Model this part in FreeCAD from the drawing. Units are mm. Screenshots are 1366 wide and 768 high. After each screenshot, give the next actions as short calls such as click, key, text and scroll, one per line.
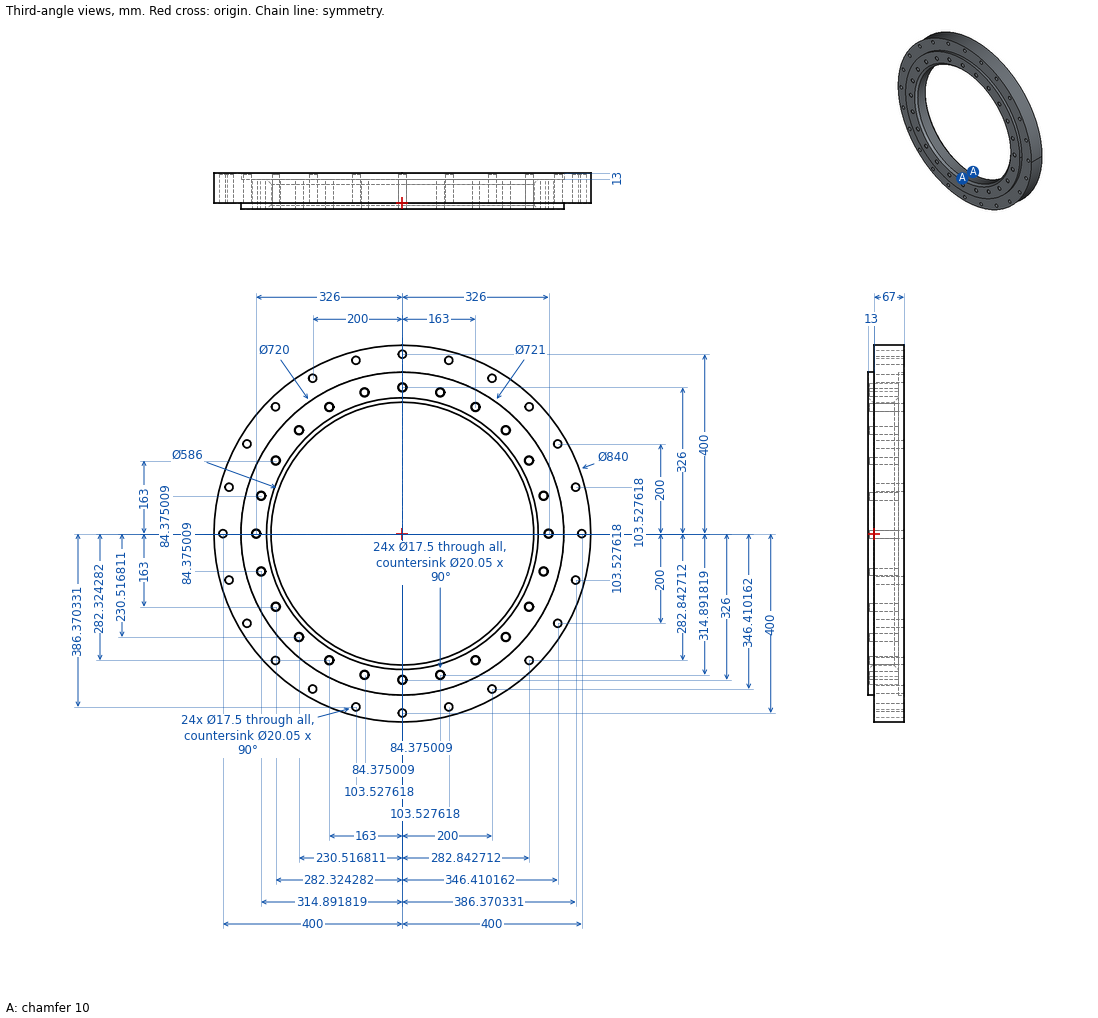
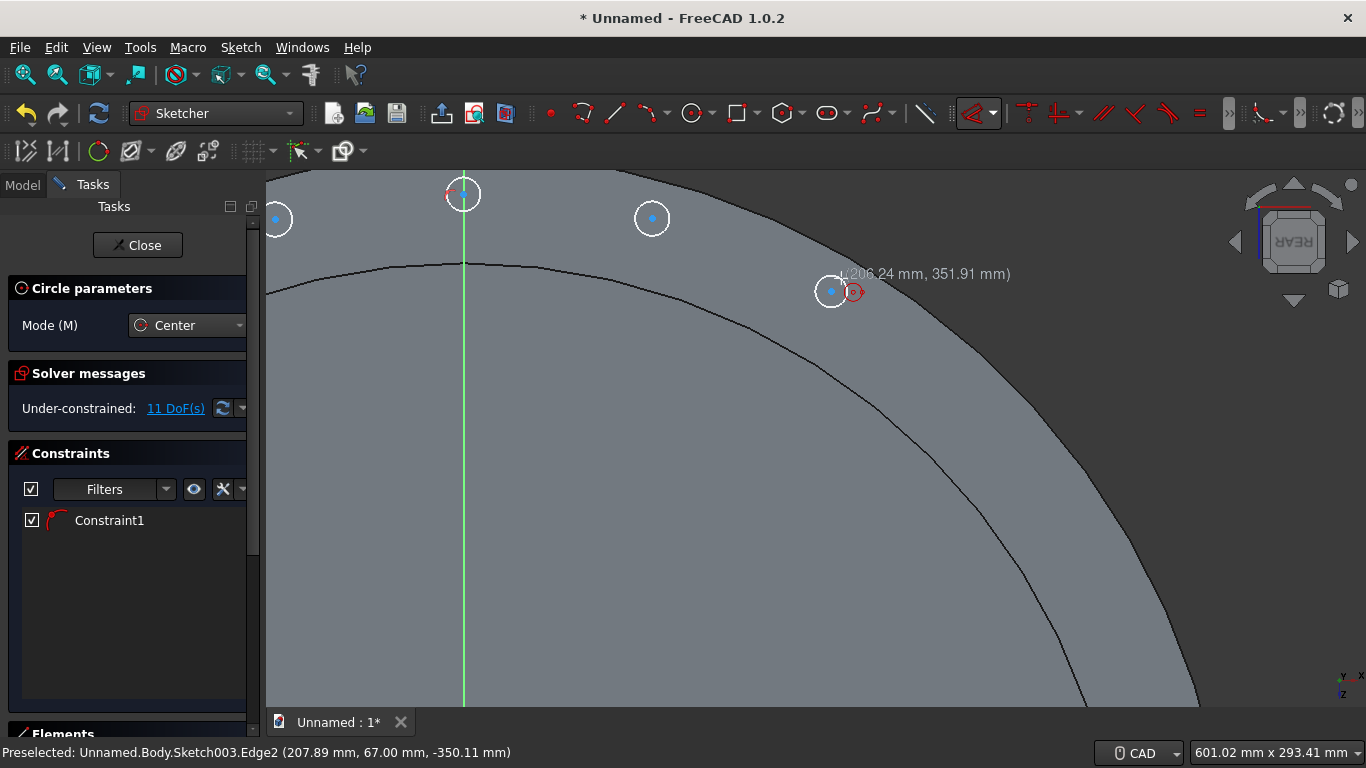
scroll(981, 405, up, 2)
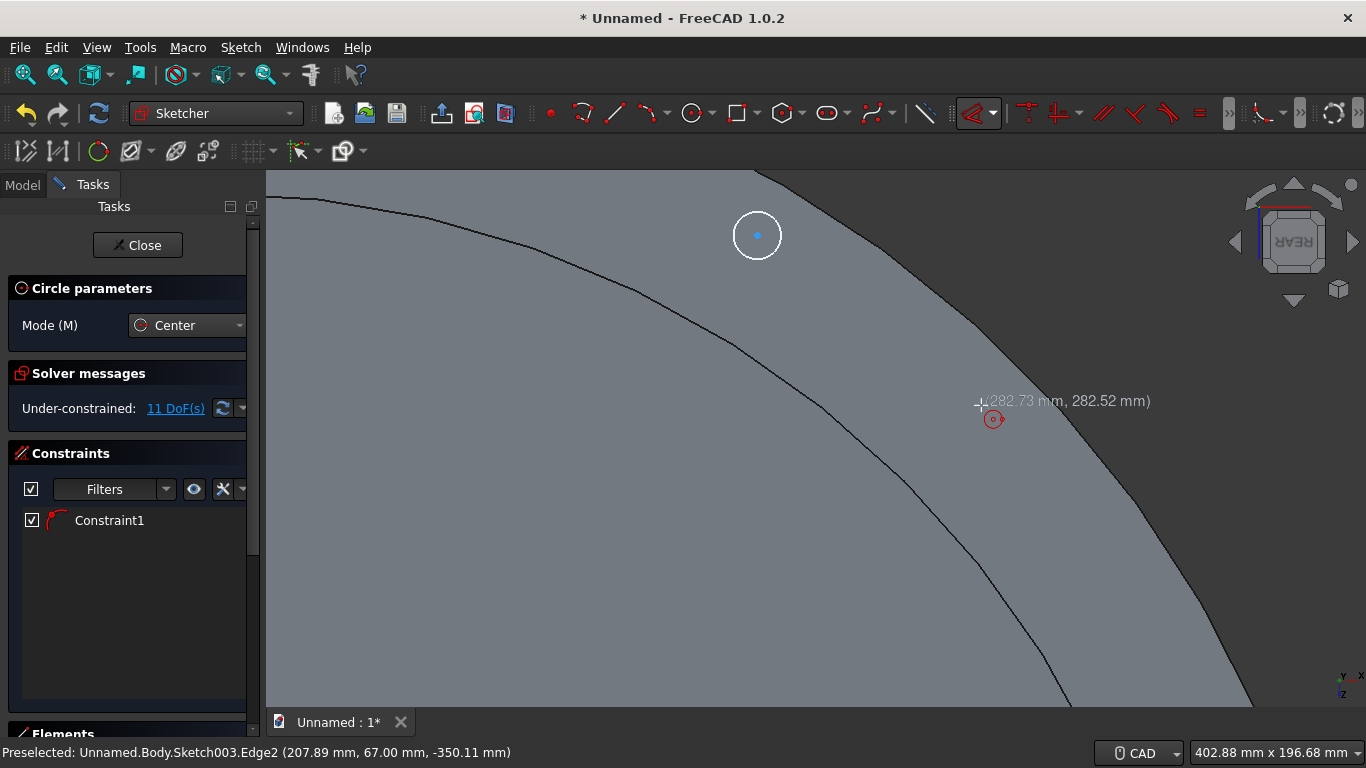
scroll(854, 292, down, 9)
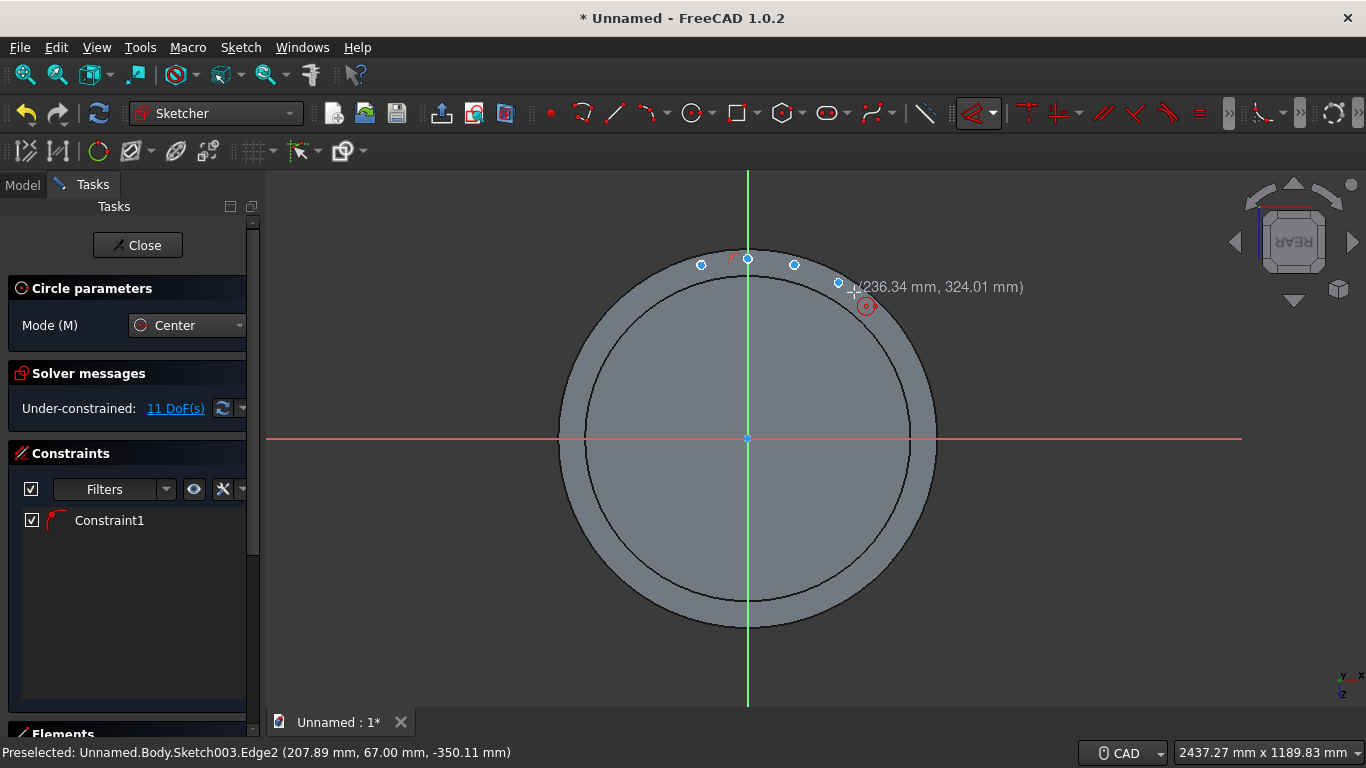
click(875, 311)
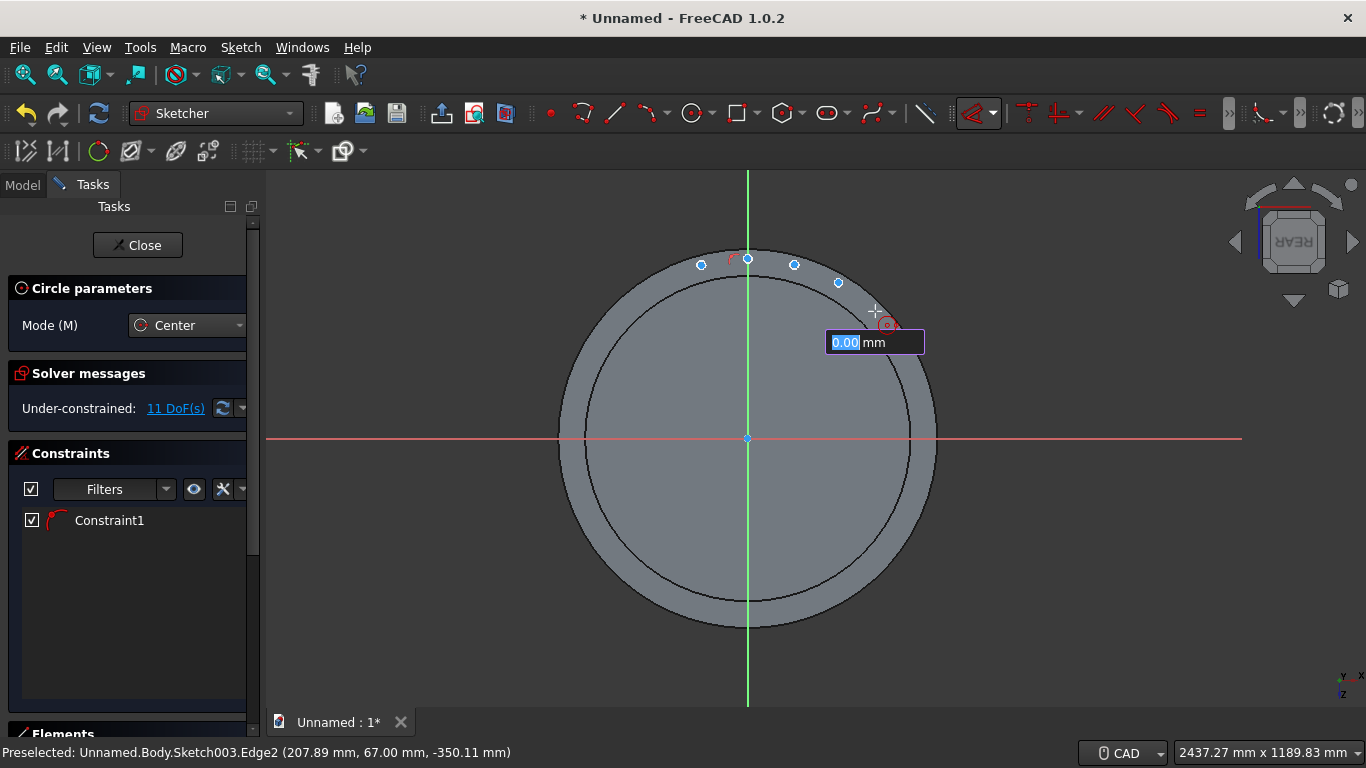
scroll(878, 308, up, 7)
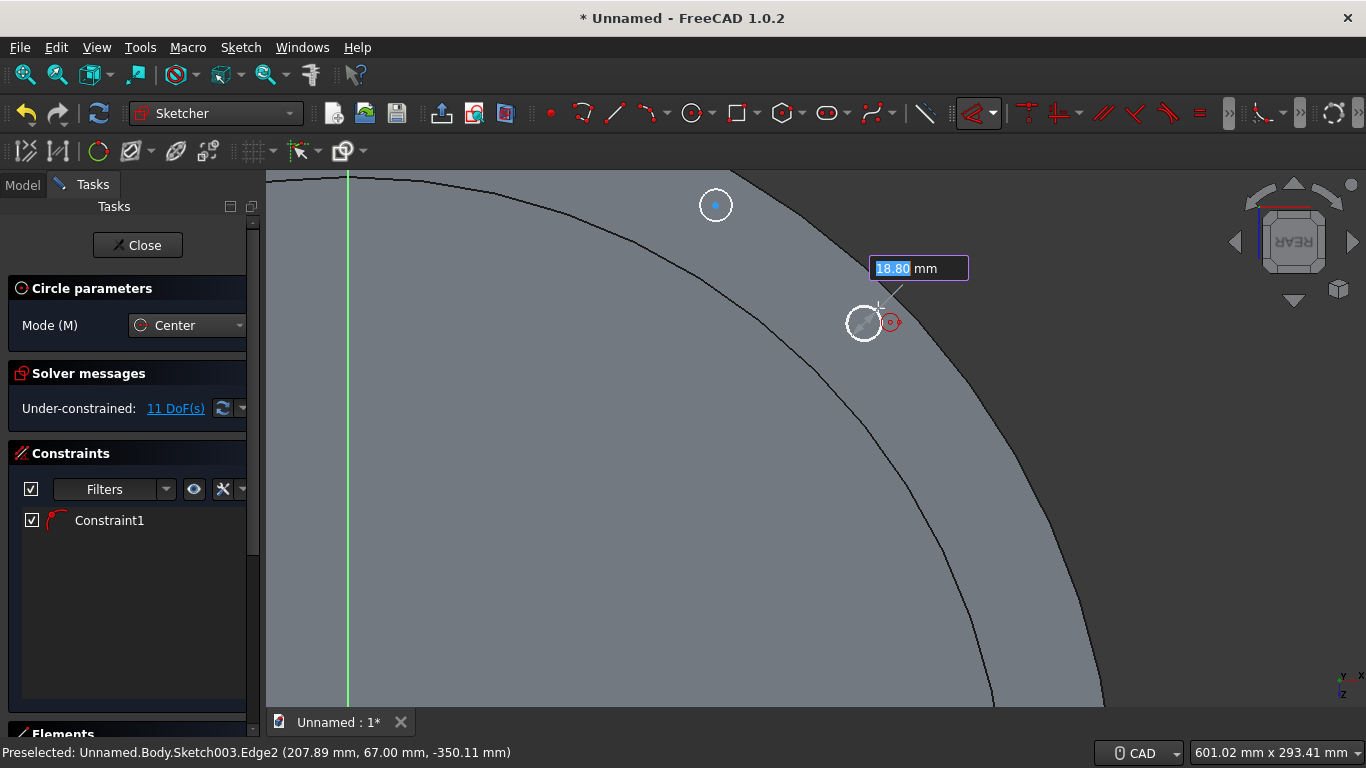
click(877, 308)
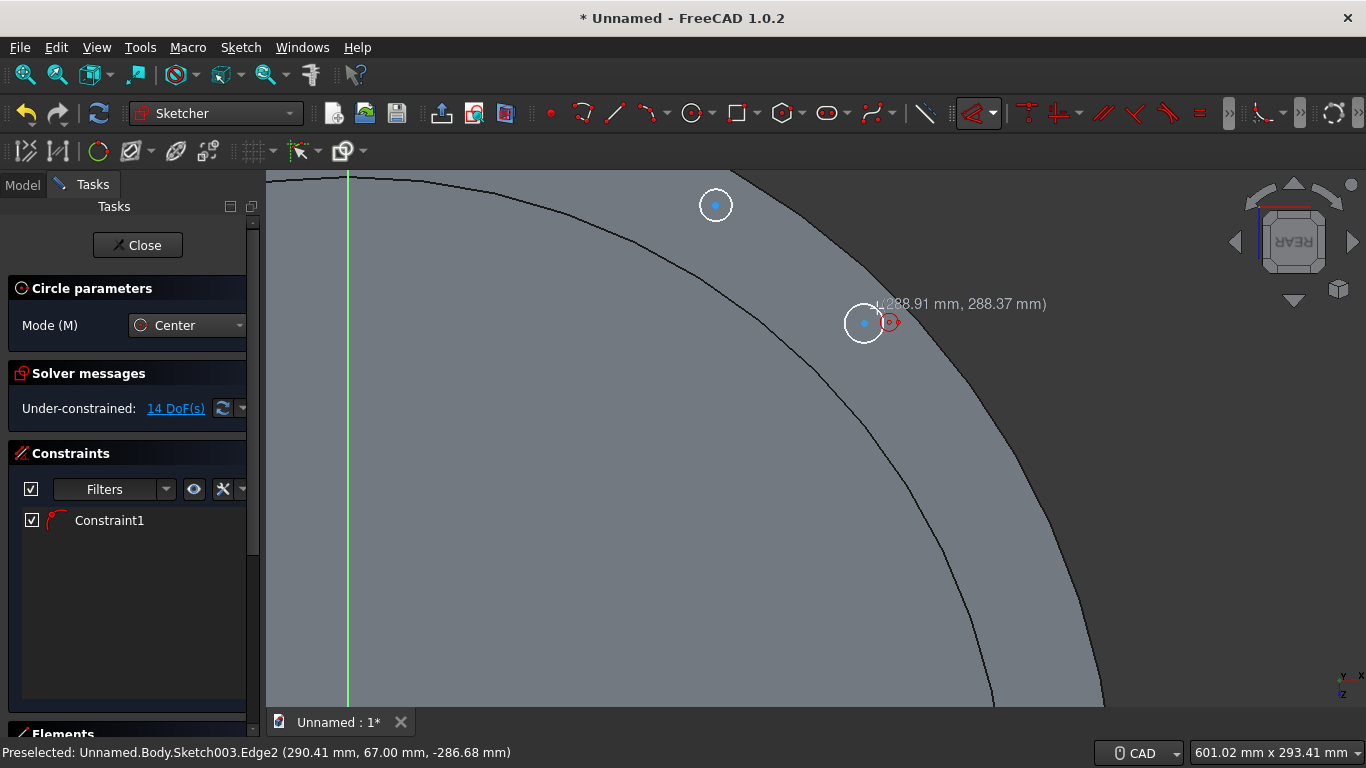
scroll(982, 471, up, 2)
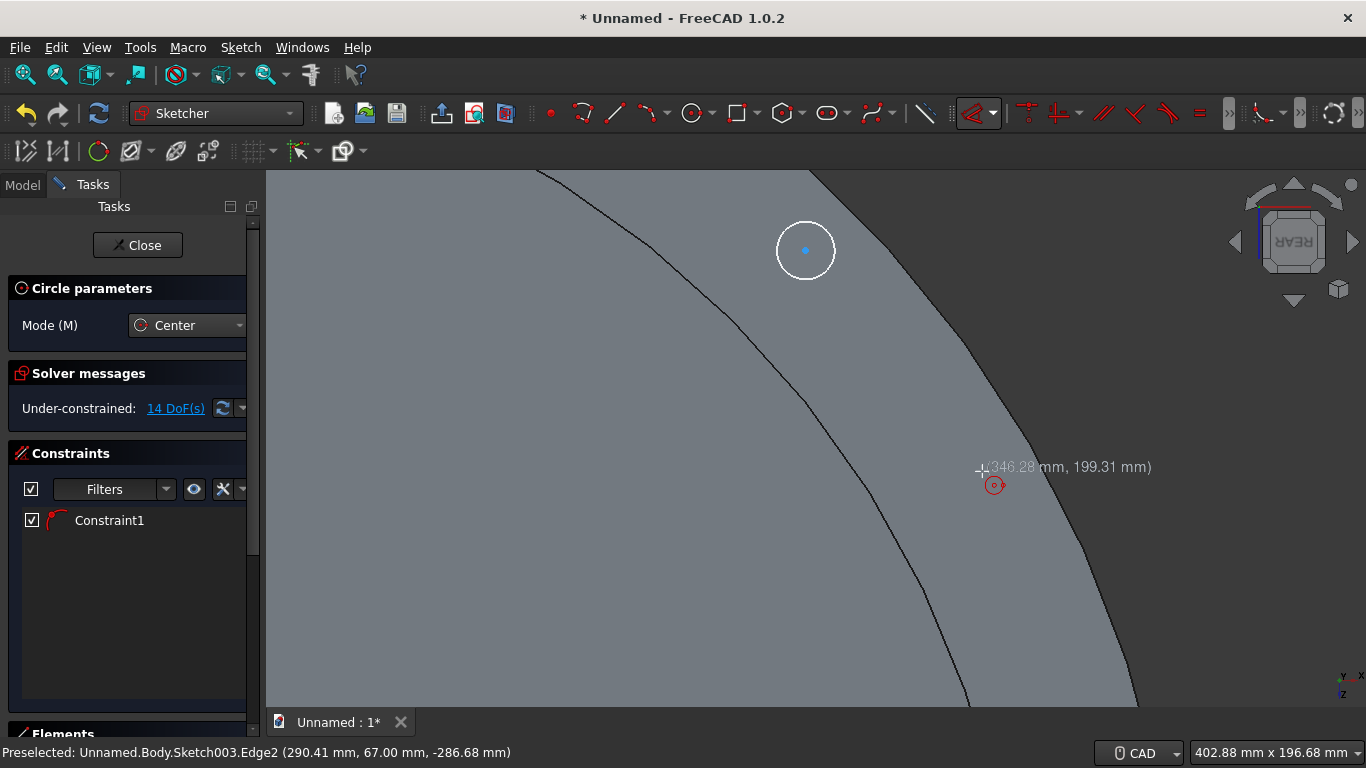
scroll(888, 324, down, 9)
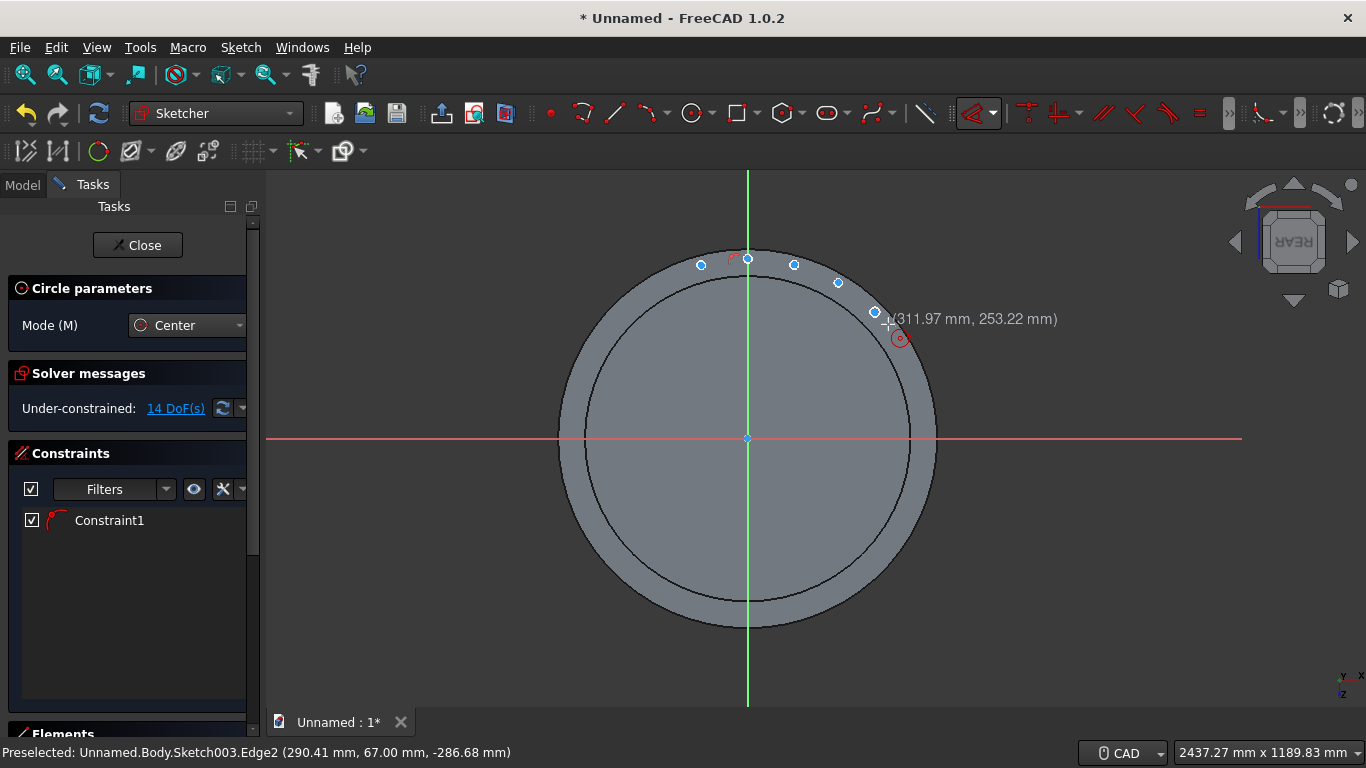
click(904, 348)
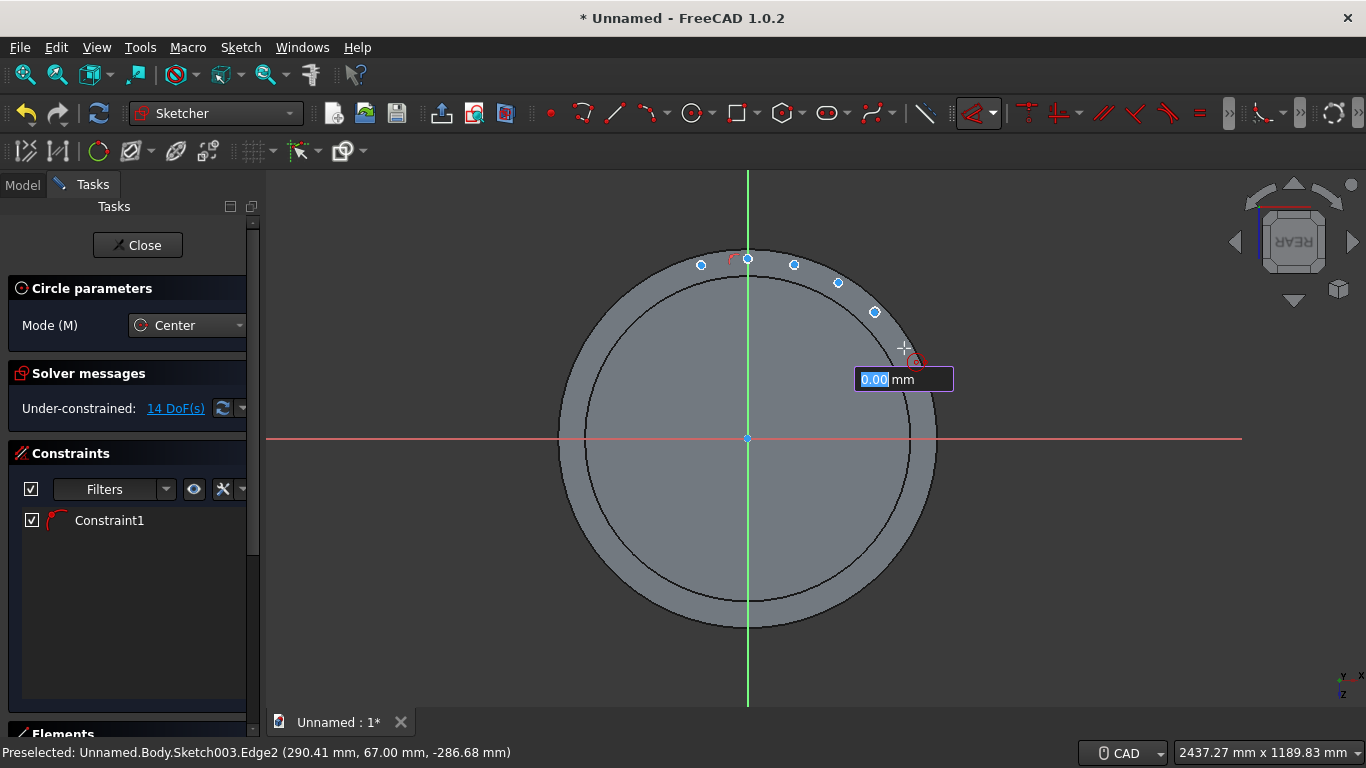
scroll(907, 346, up, 7)